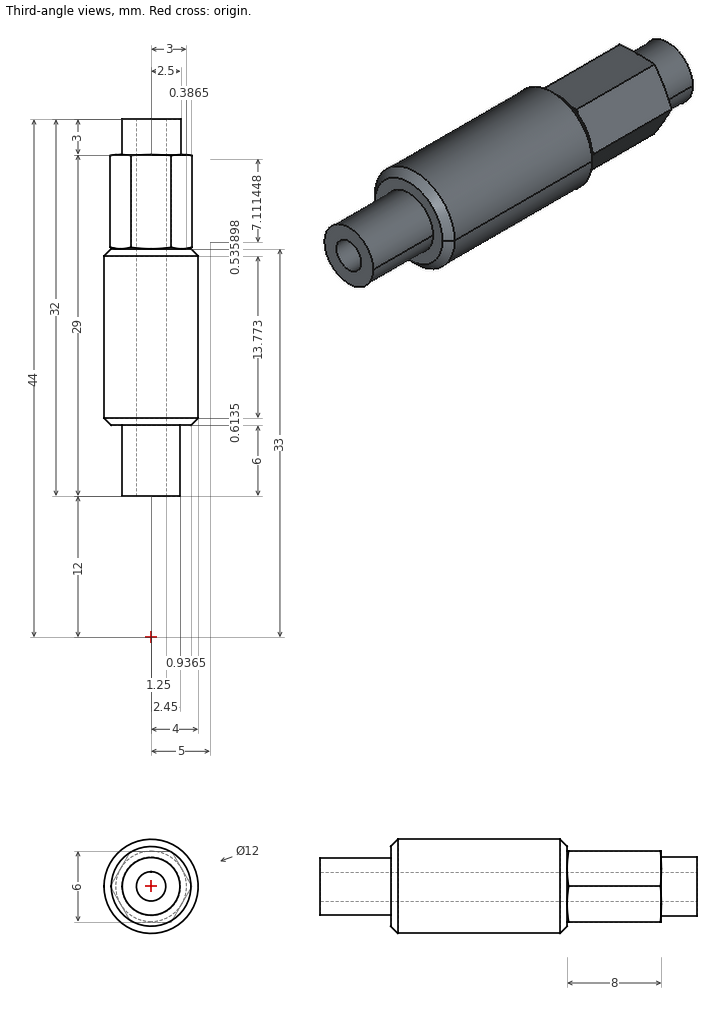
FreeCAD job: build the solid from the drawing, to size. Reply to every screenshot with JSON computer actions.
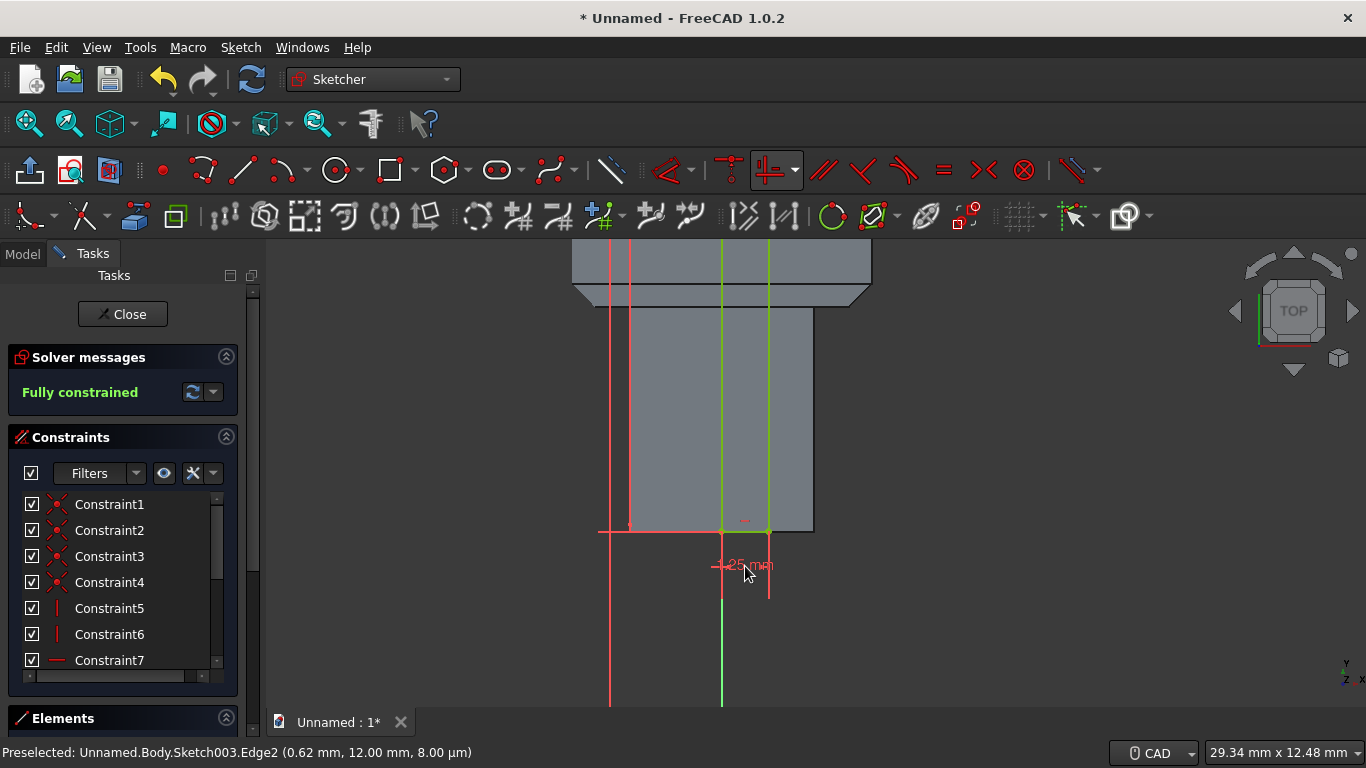
{"action": "left_click", "coordinate": [123, 314]}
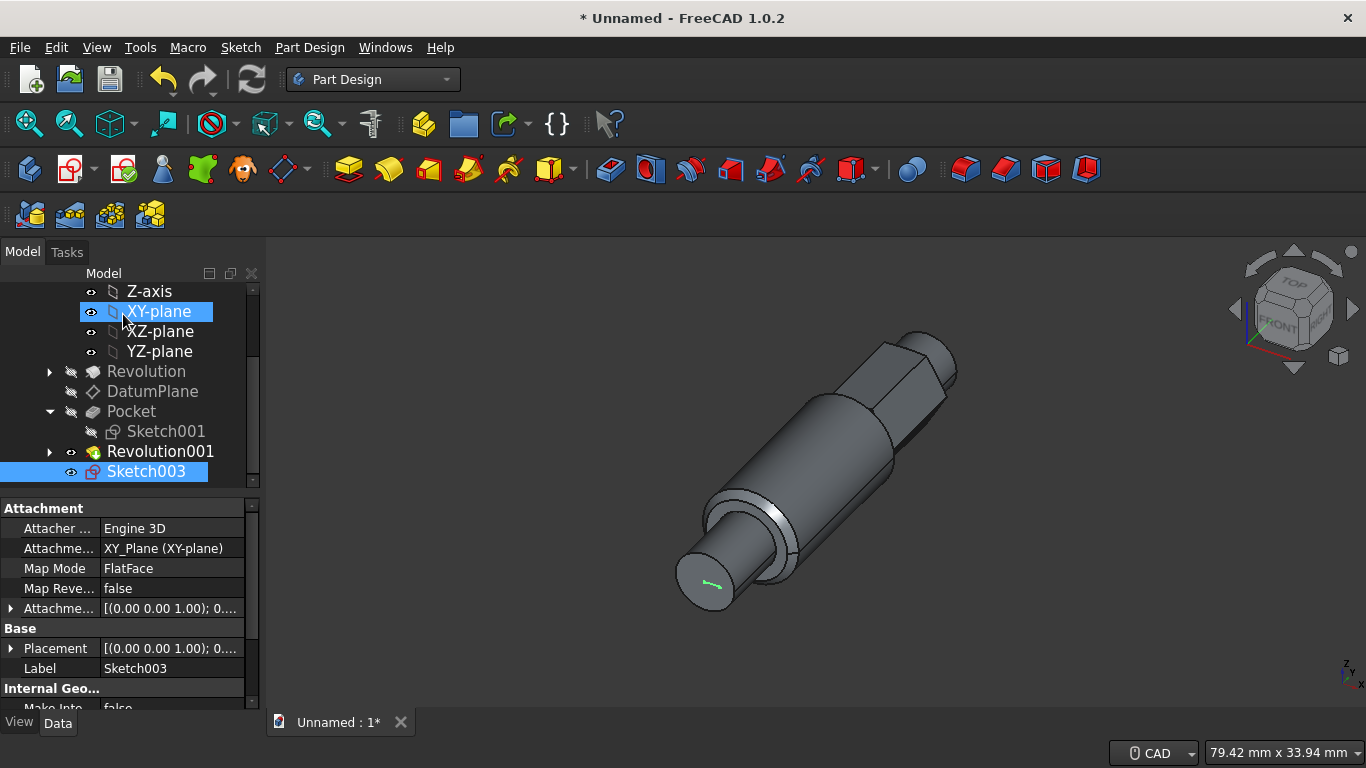
{"action": "left_click", "coordinate": [692, 170]}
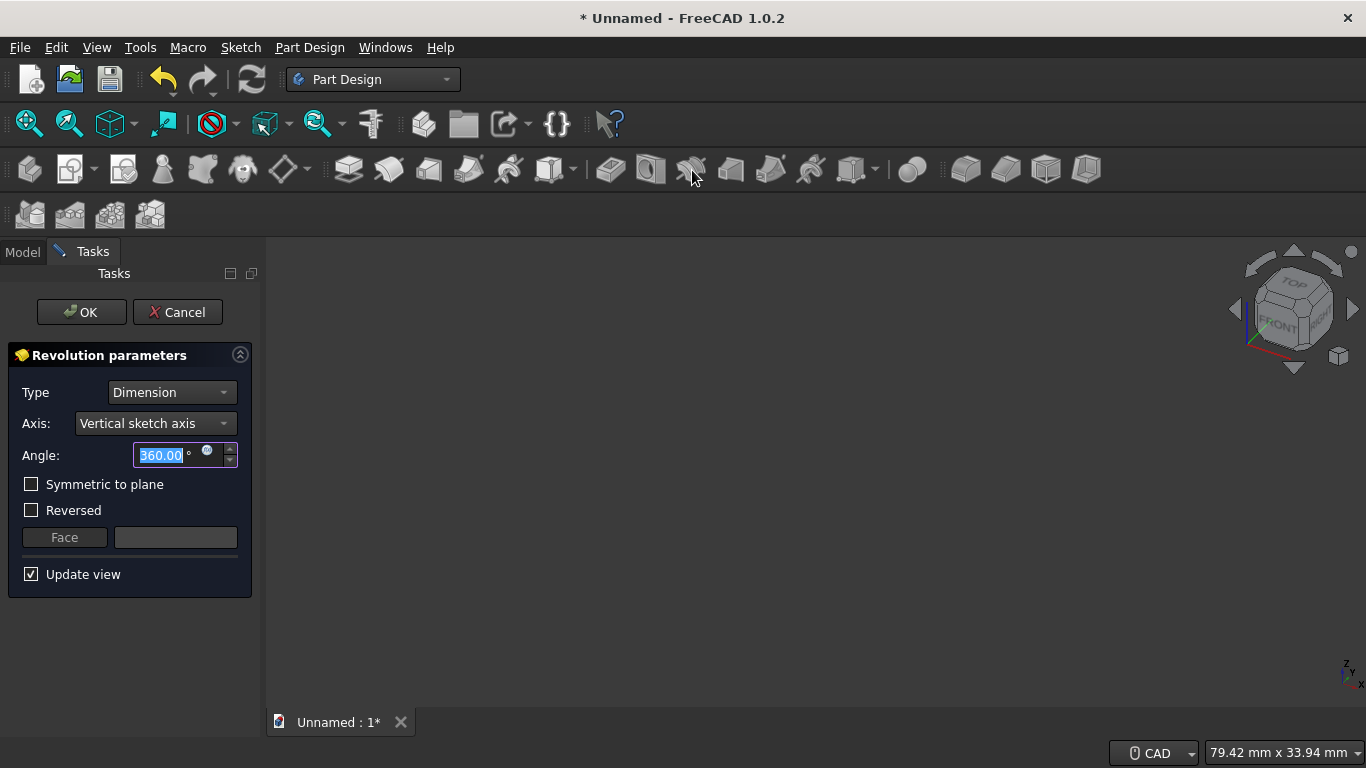
{"action": "left_click", "coordinate": [82, 312]}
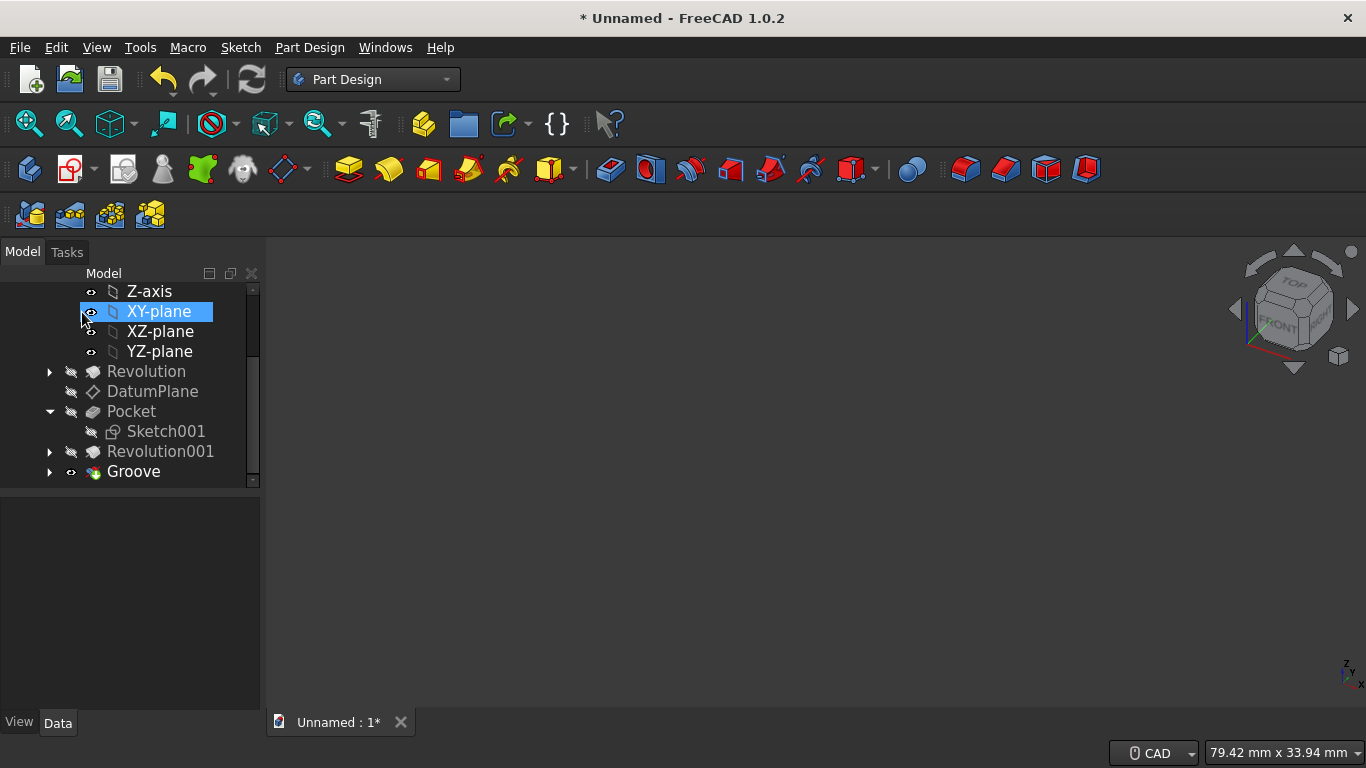
{"action": "key", "text": "0"}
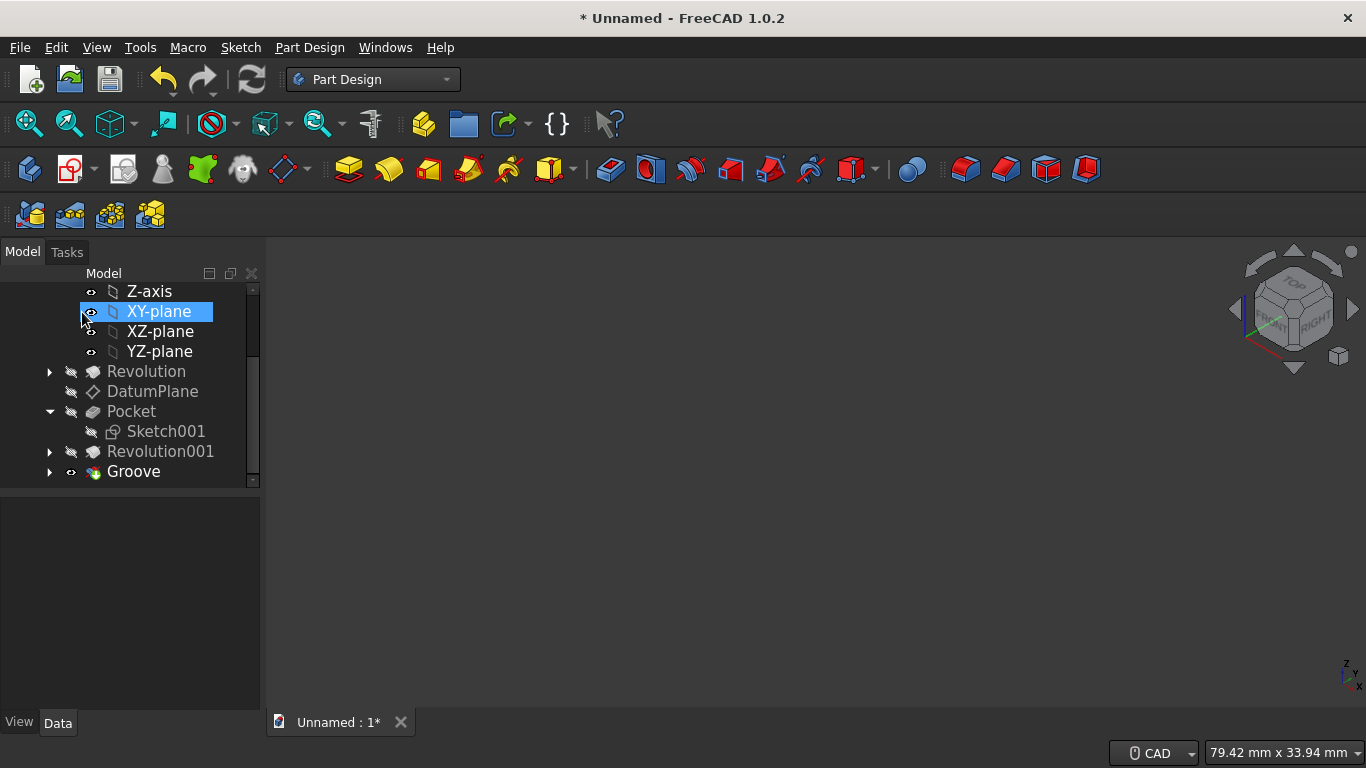
{"action": "left_click", "coordinate": [30, 124]}